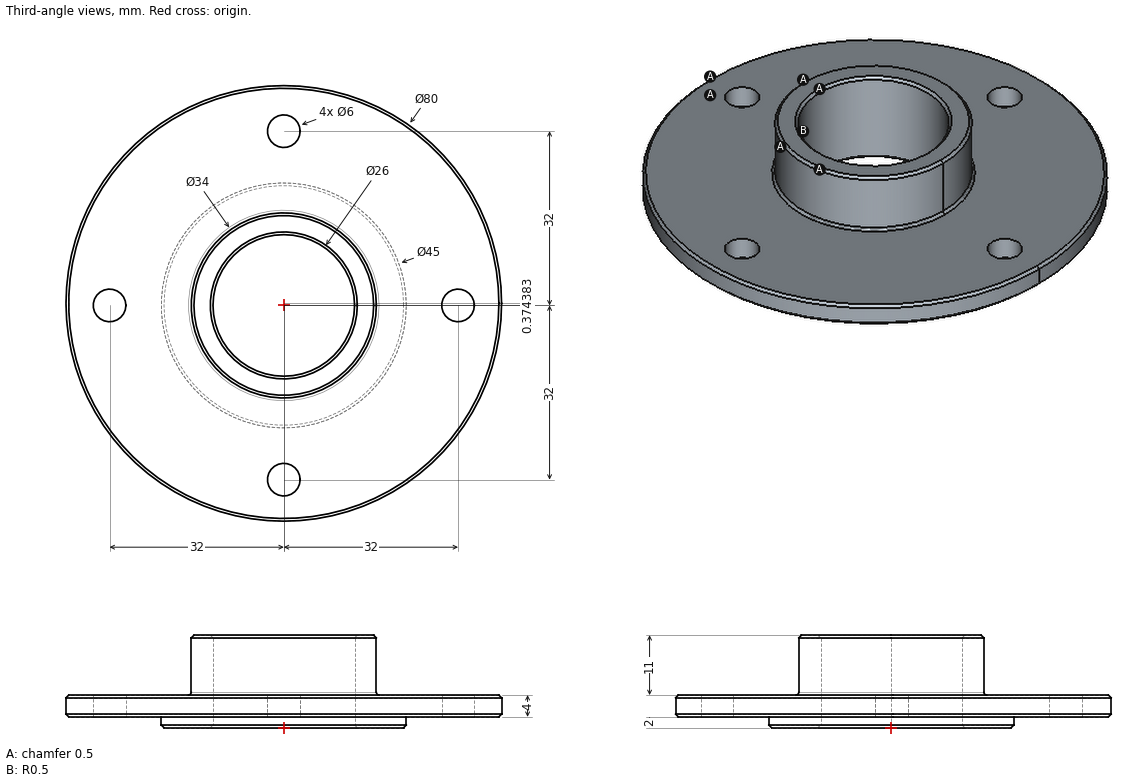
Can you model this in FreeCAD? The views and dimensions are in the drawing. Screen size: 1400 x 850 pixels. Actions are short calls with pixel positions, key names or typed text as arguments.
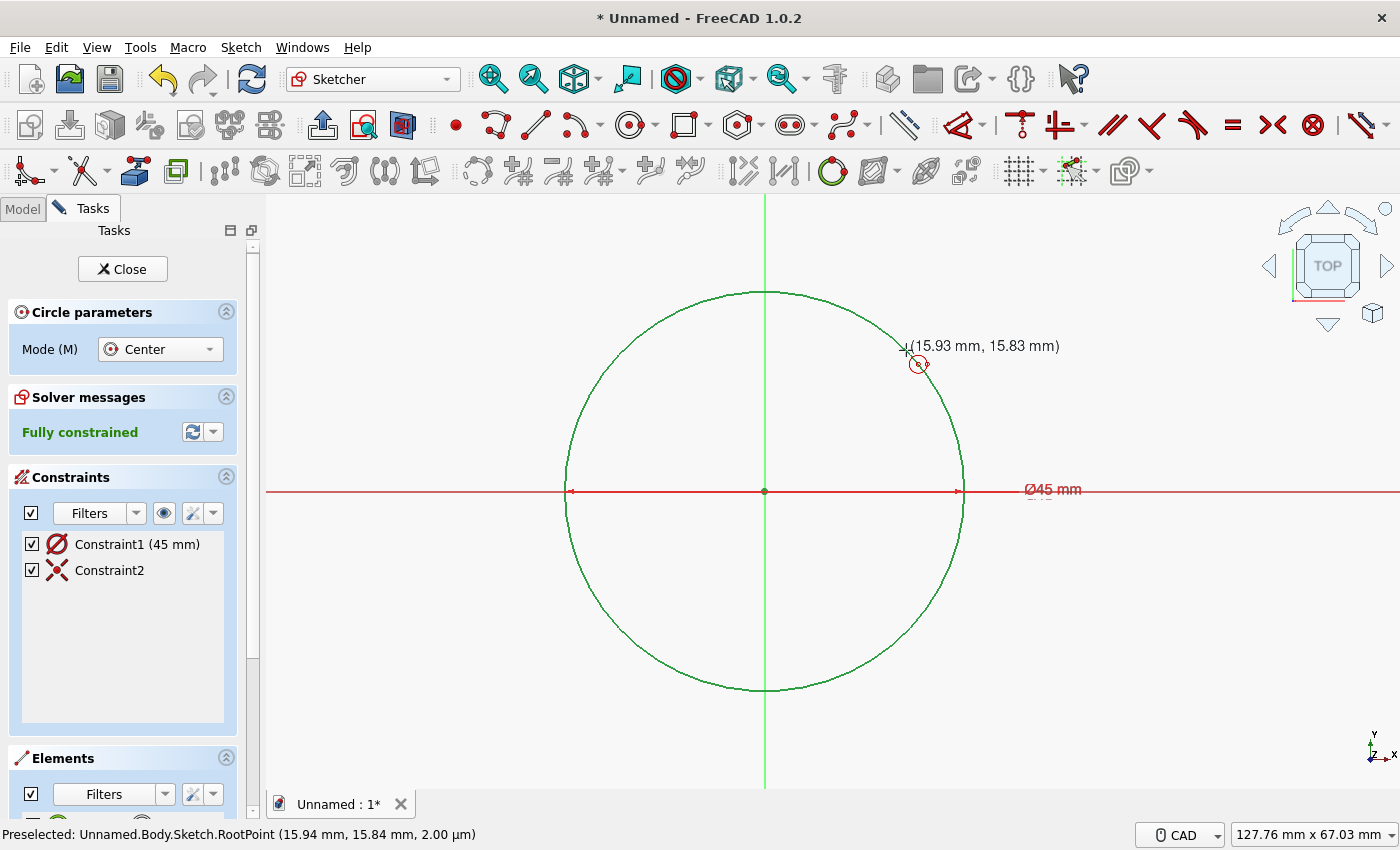
click(765, 492)
move(846, 410)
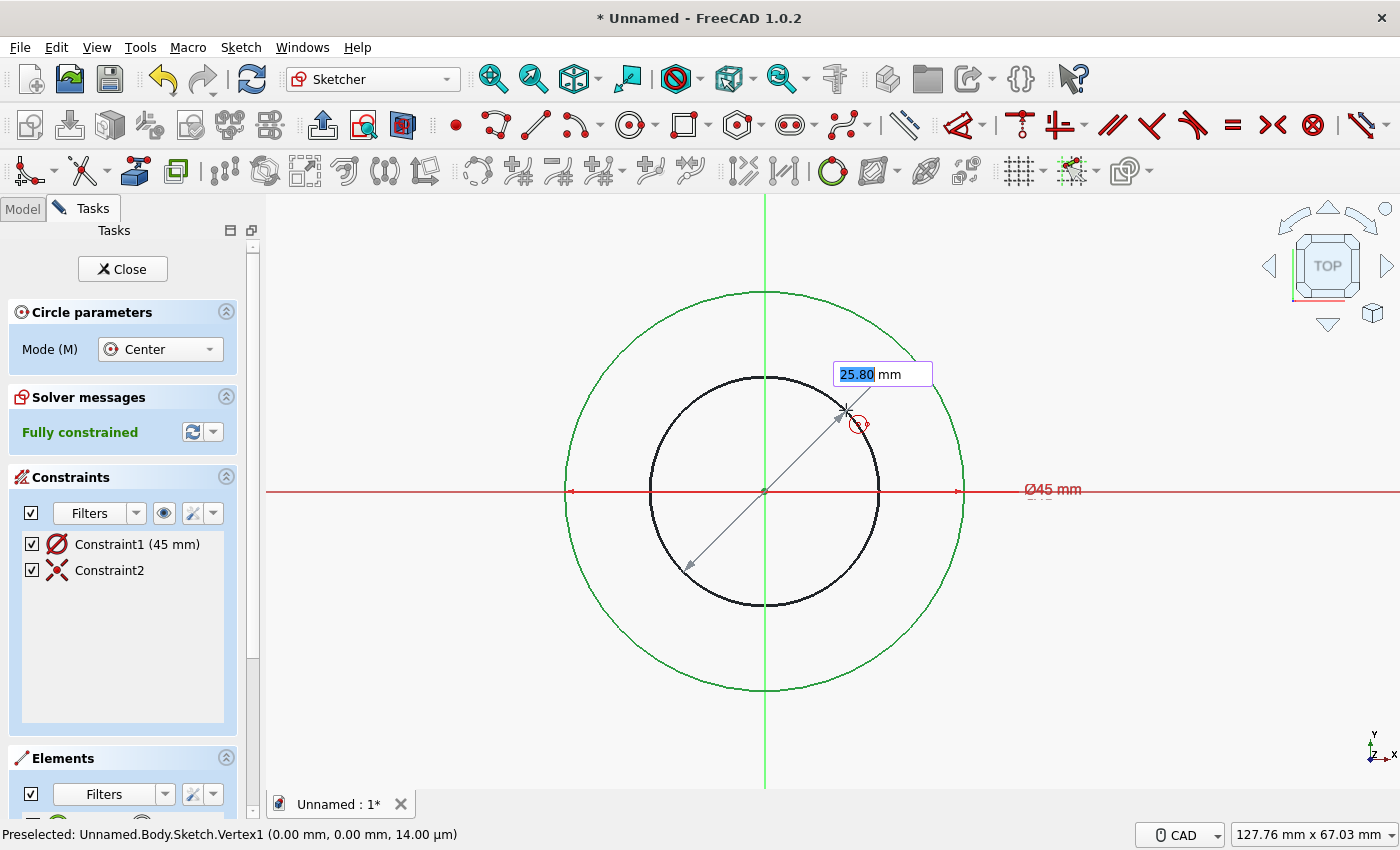
text(26)
key(Return)
key(Escape)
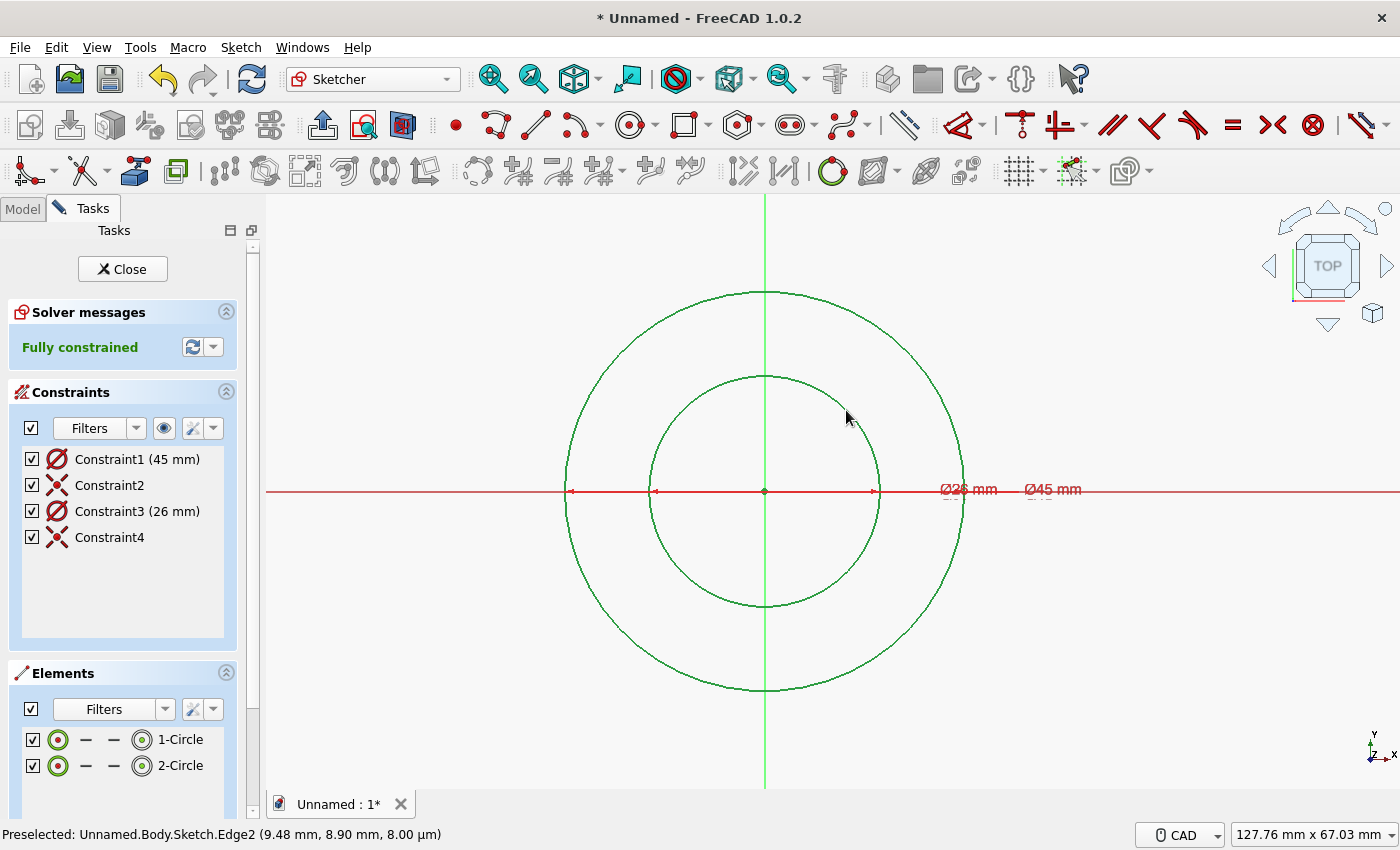
click(123, 269)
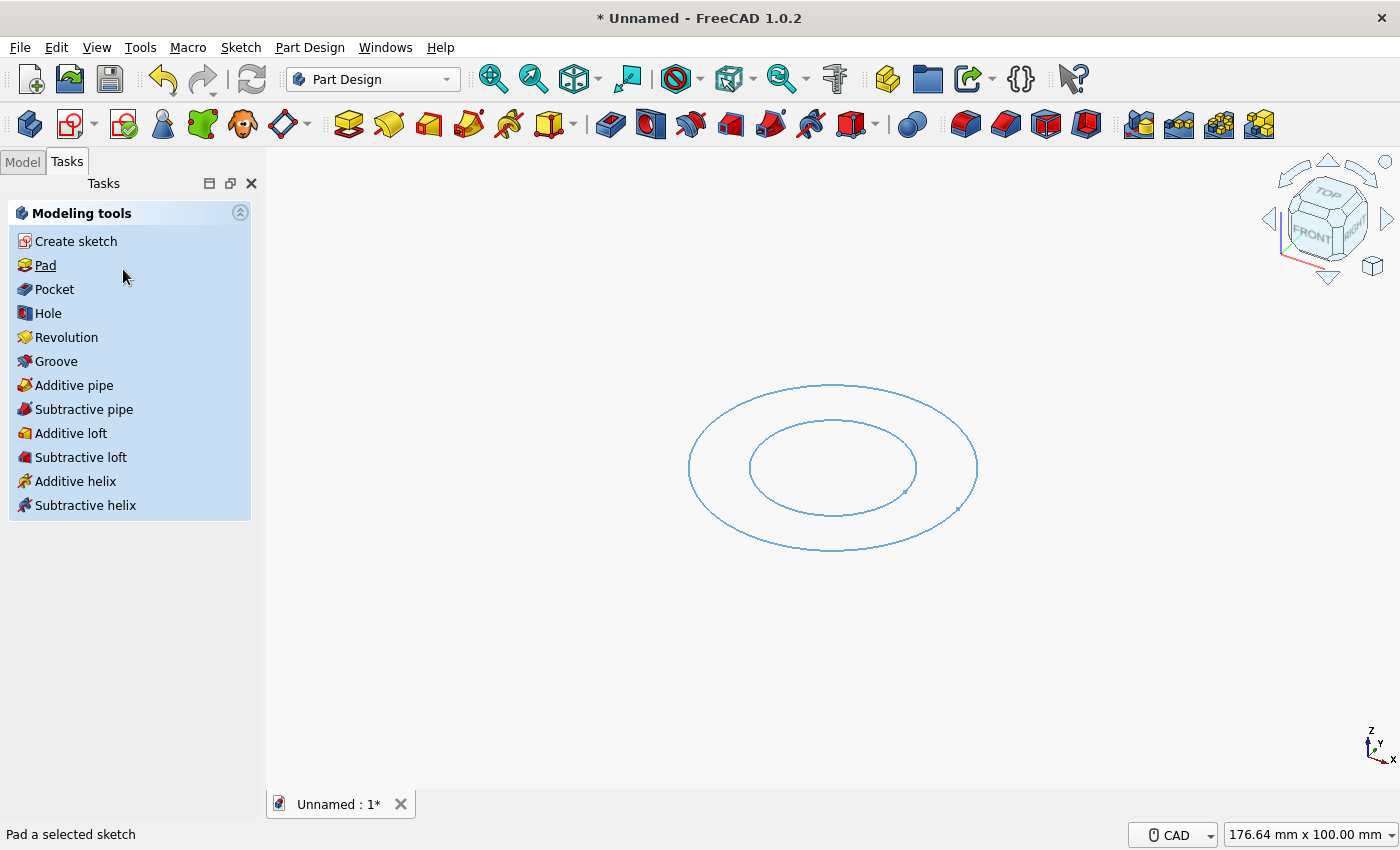
click(350, 124)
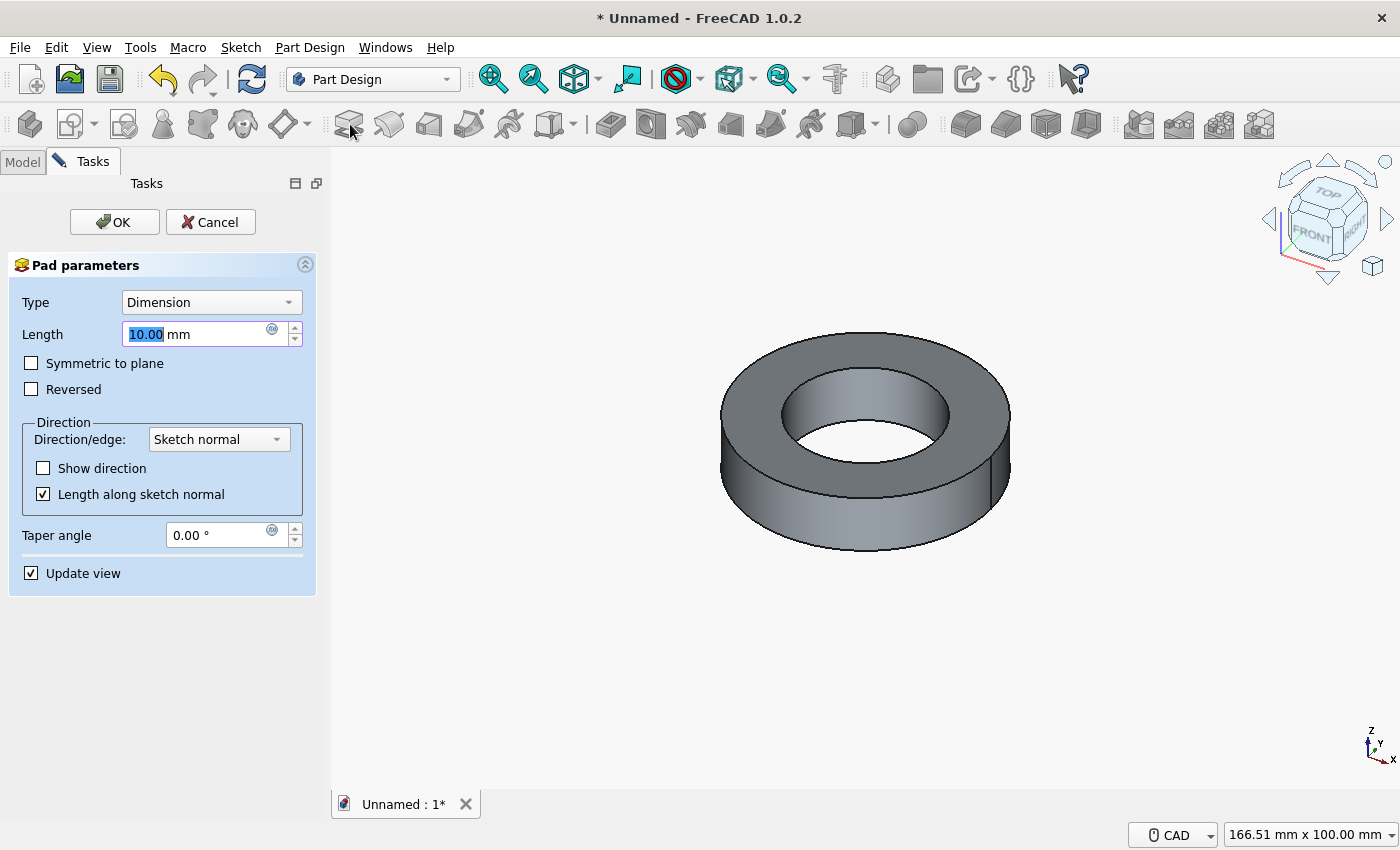
text(2)
key(Tab)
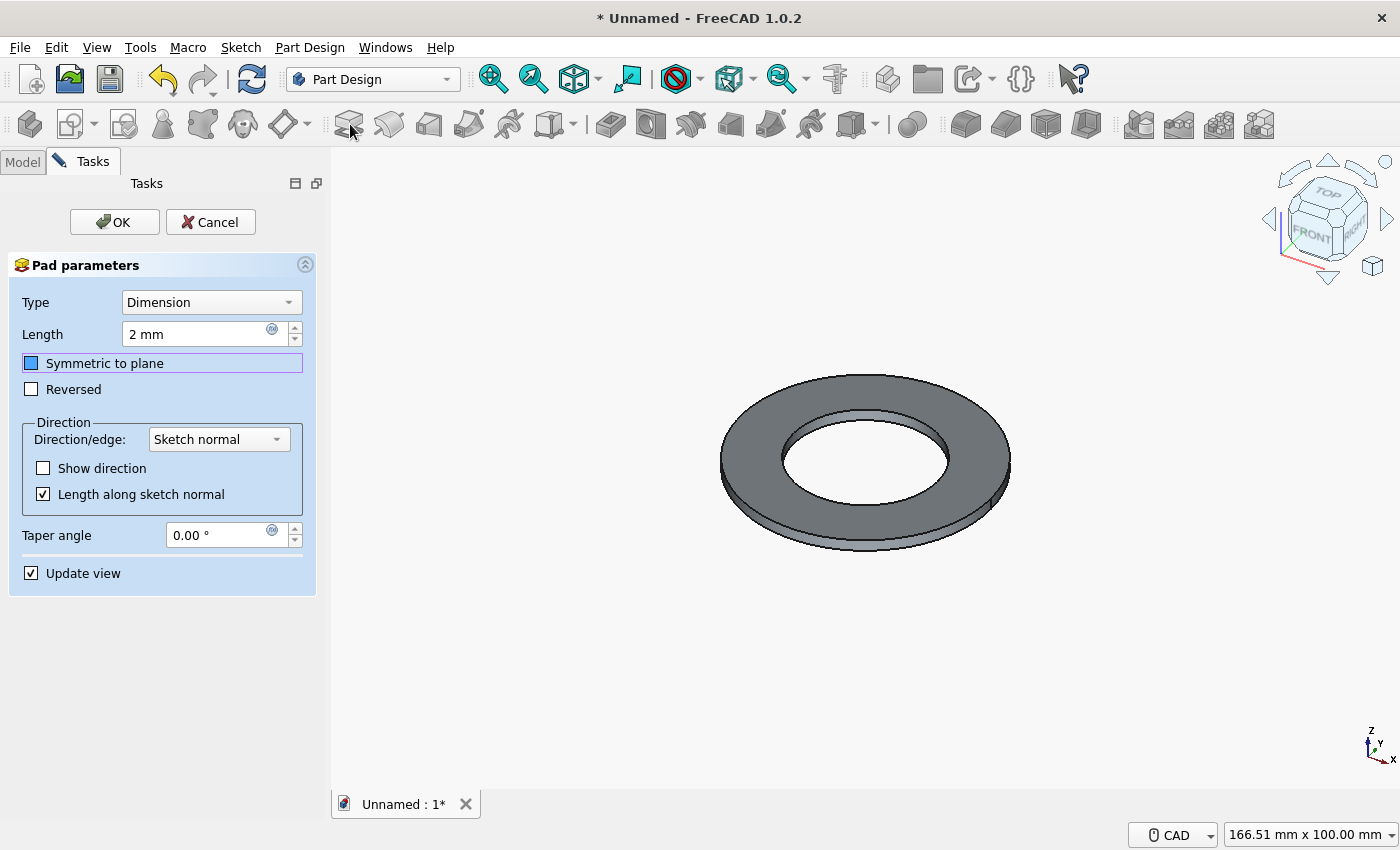
click(115, 222)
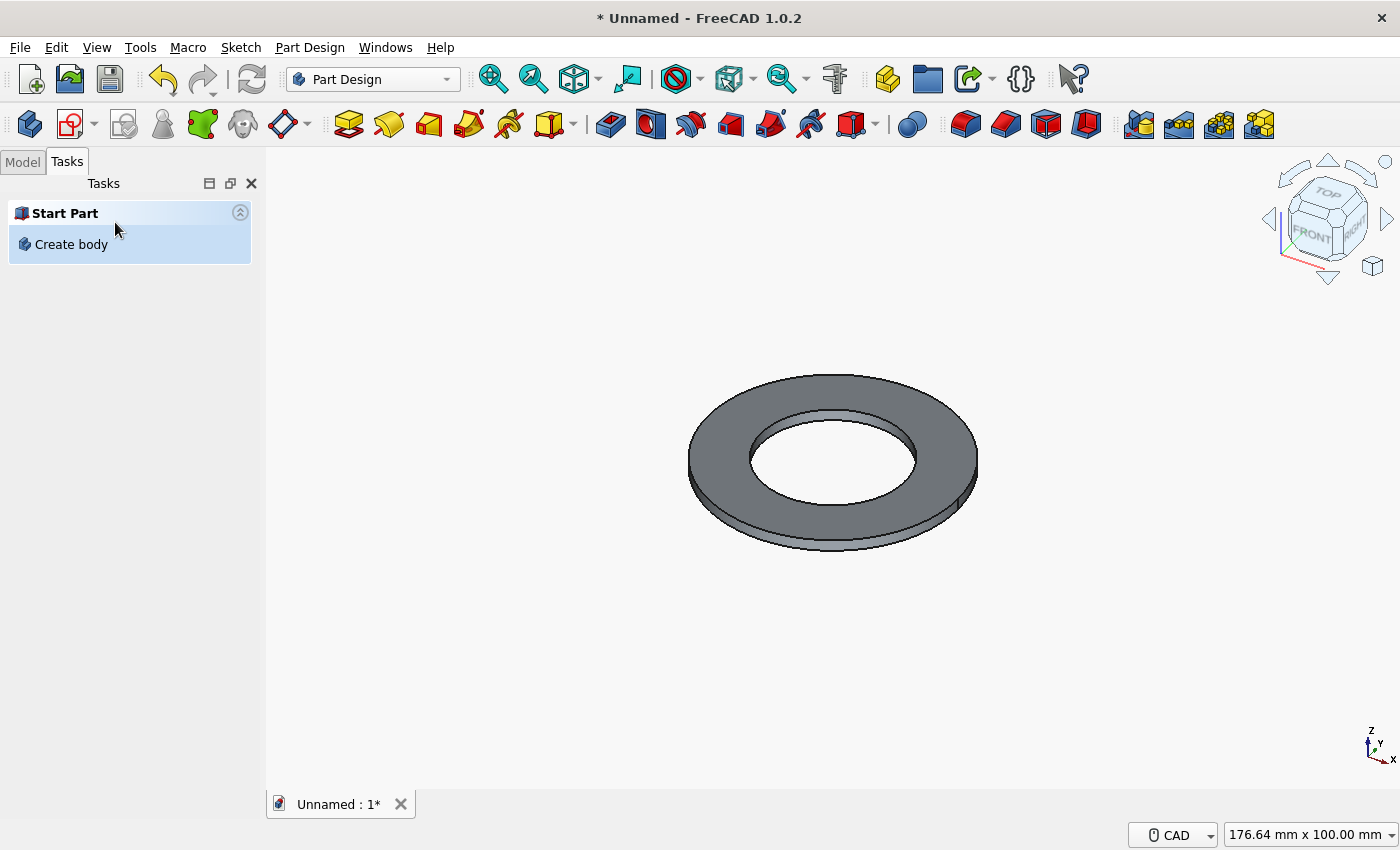
click(494, 80)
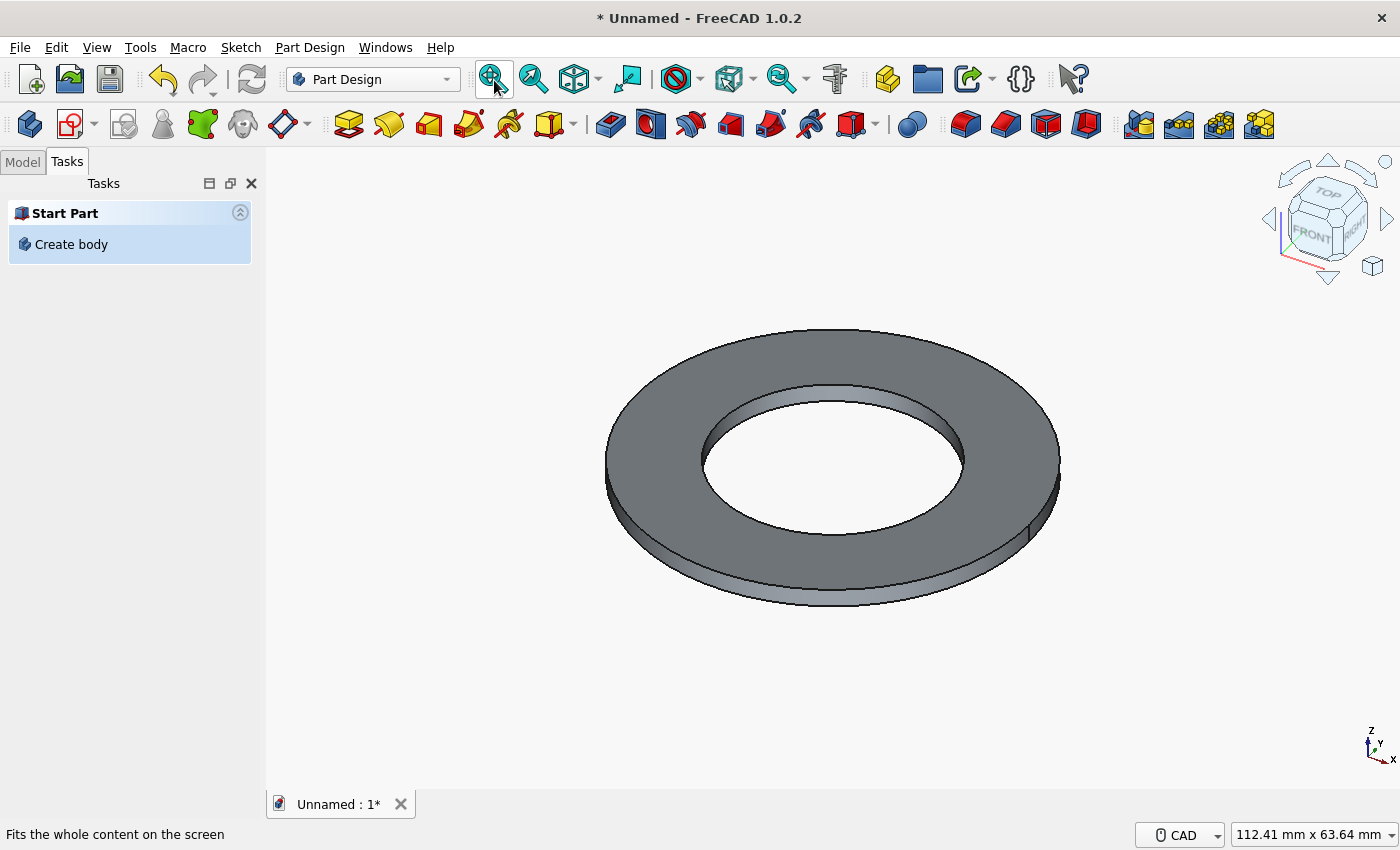
click(1010, 431)